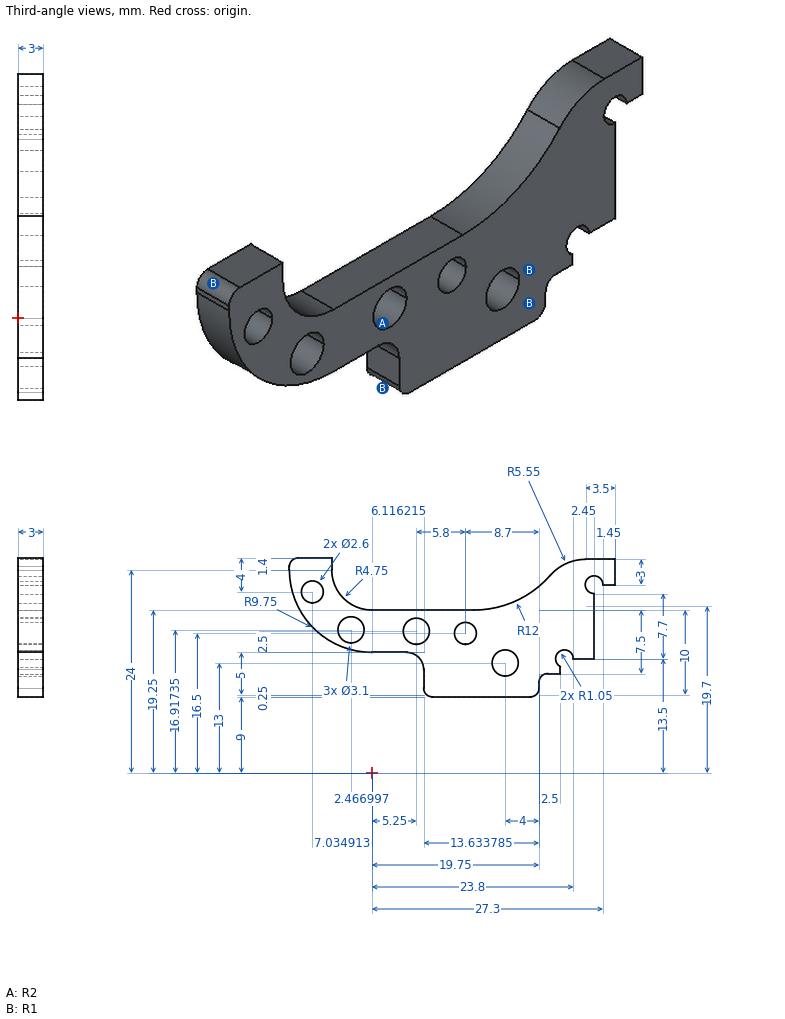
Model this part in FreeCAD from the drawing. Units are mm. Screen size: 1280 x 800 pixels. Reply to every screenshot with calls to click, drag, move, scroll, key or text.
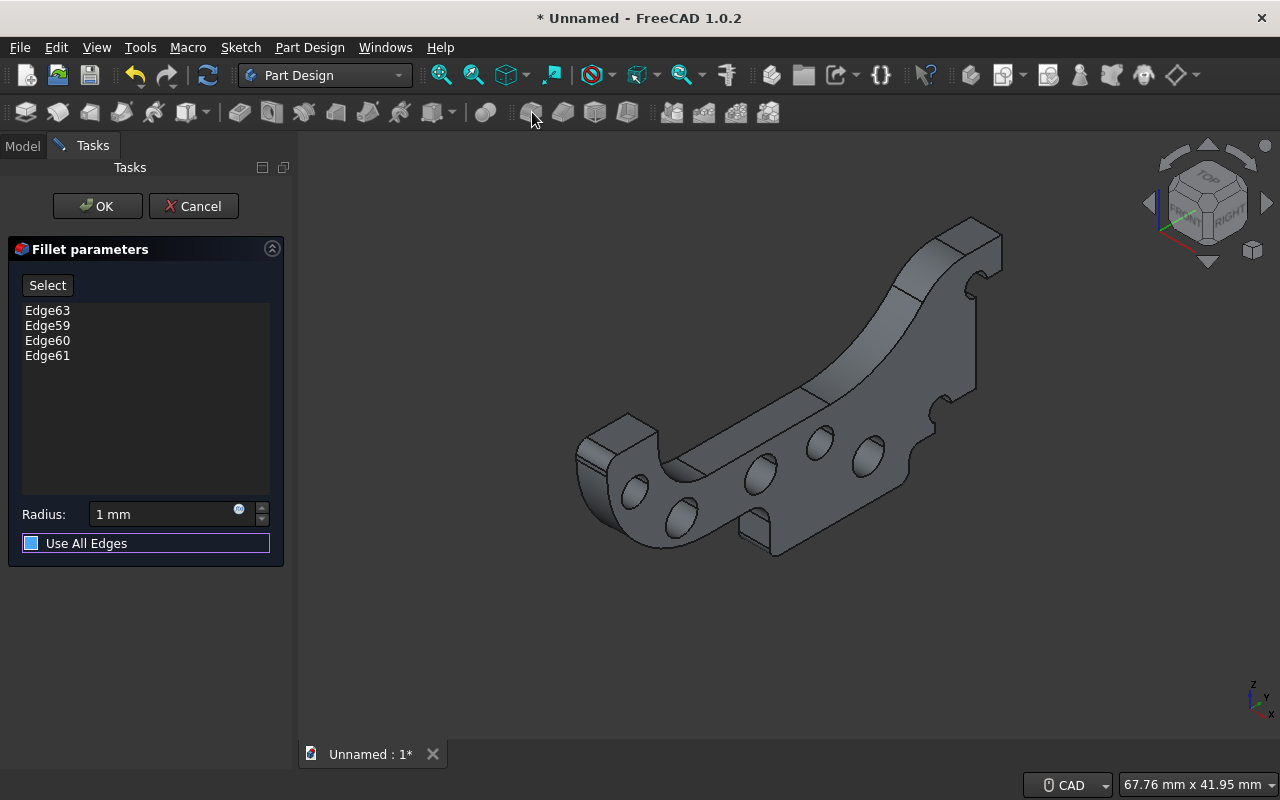
click(98, 206)